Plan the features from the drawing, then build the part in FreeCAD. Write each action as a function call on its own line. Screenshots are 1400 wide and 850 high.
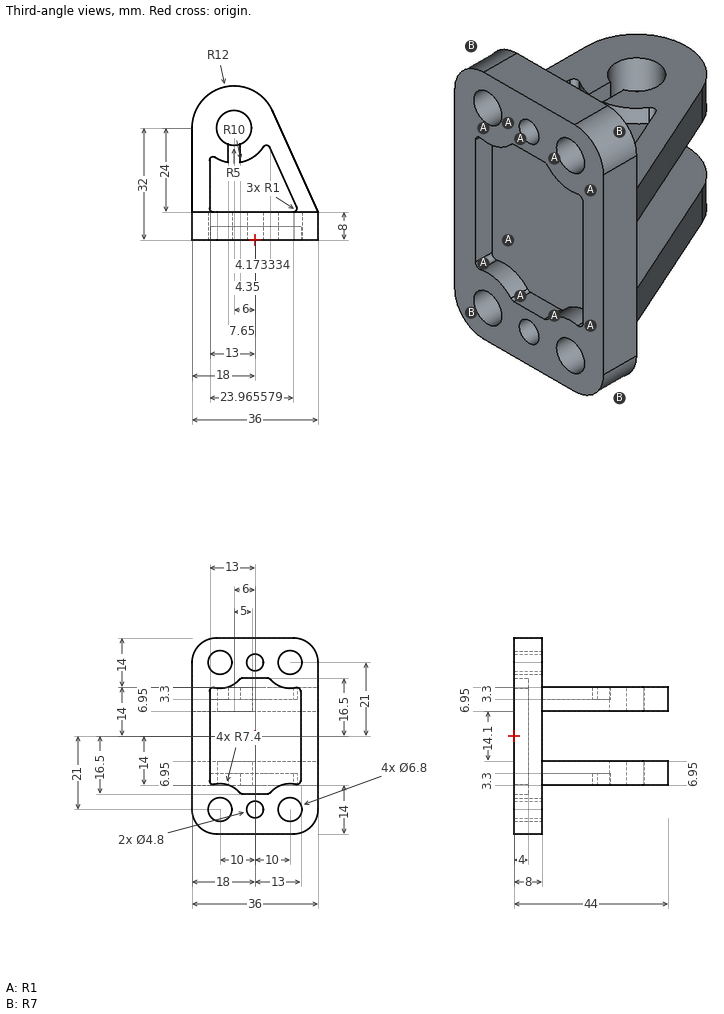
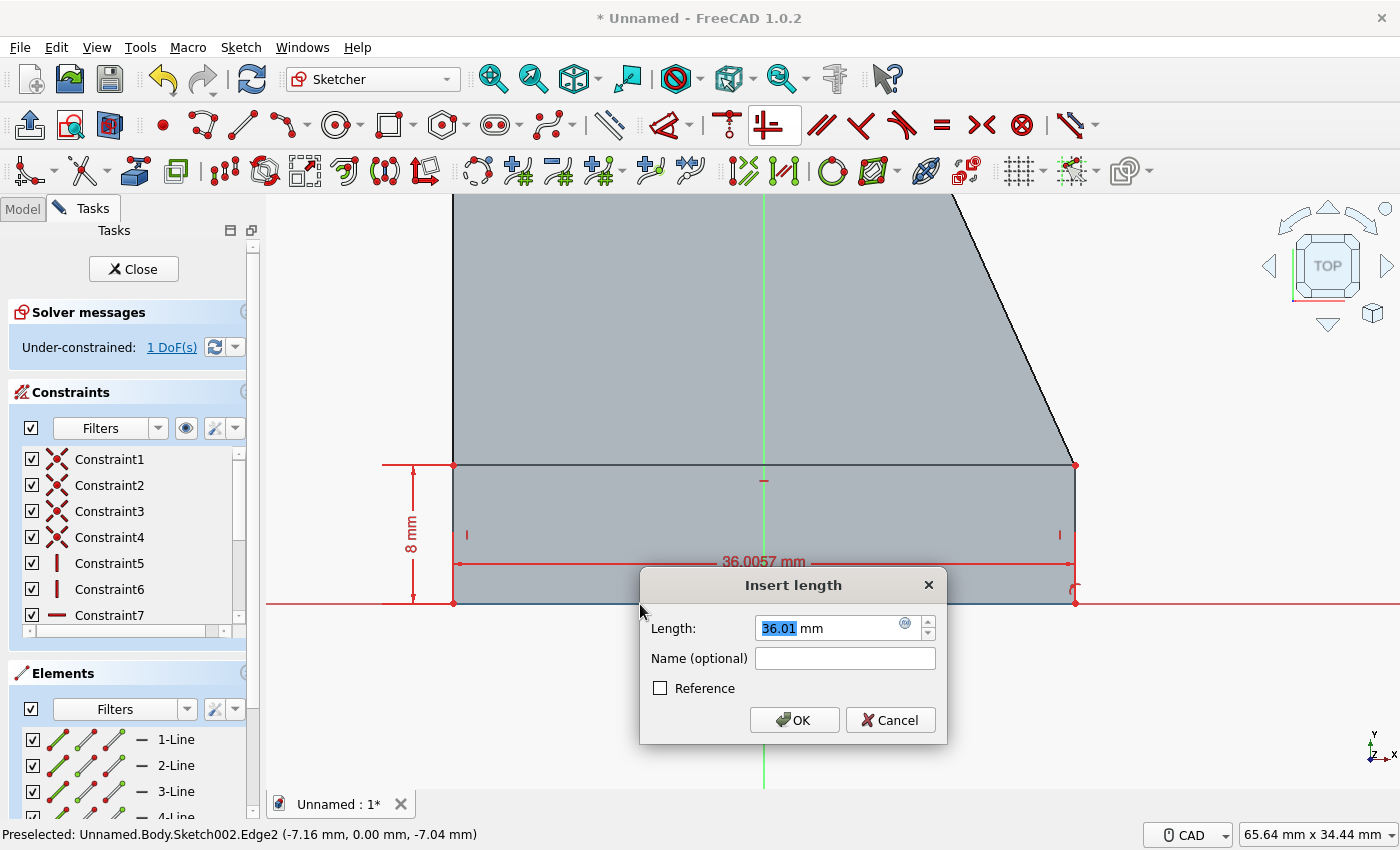
text(36)
key(Return)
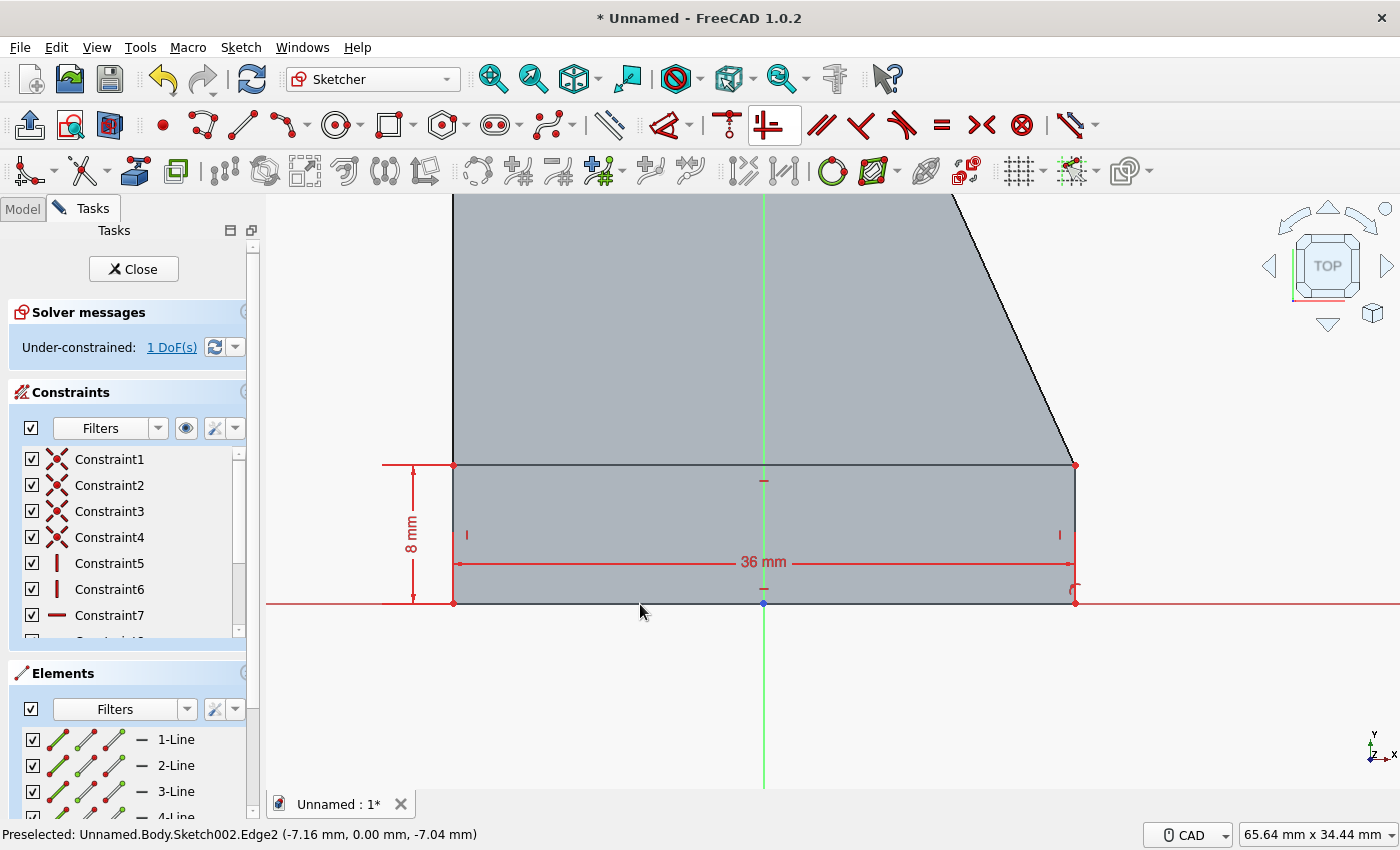
click(453, 465)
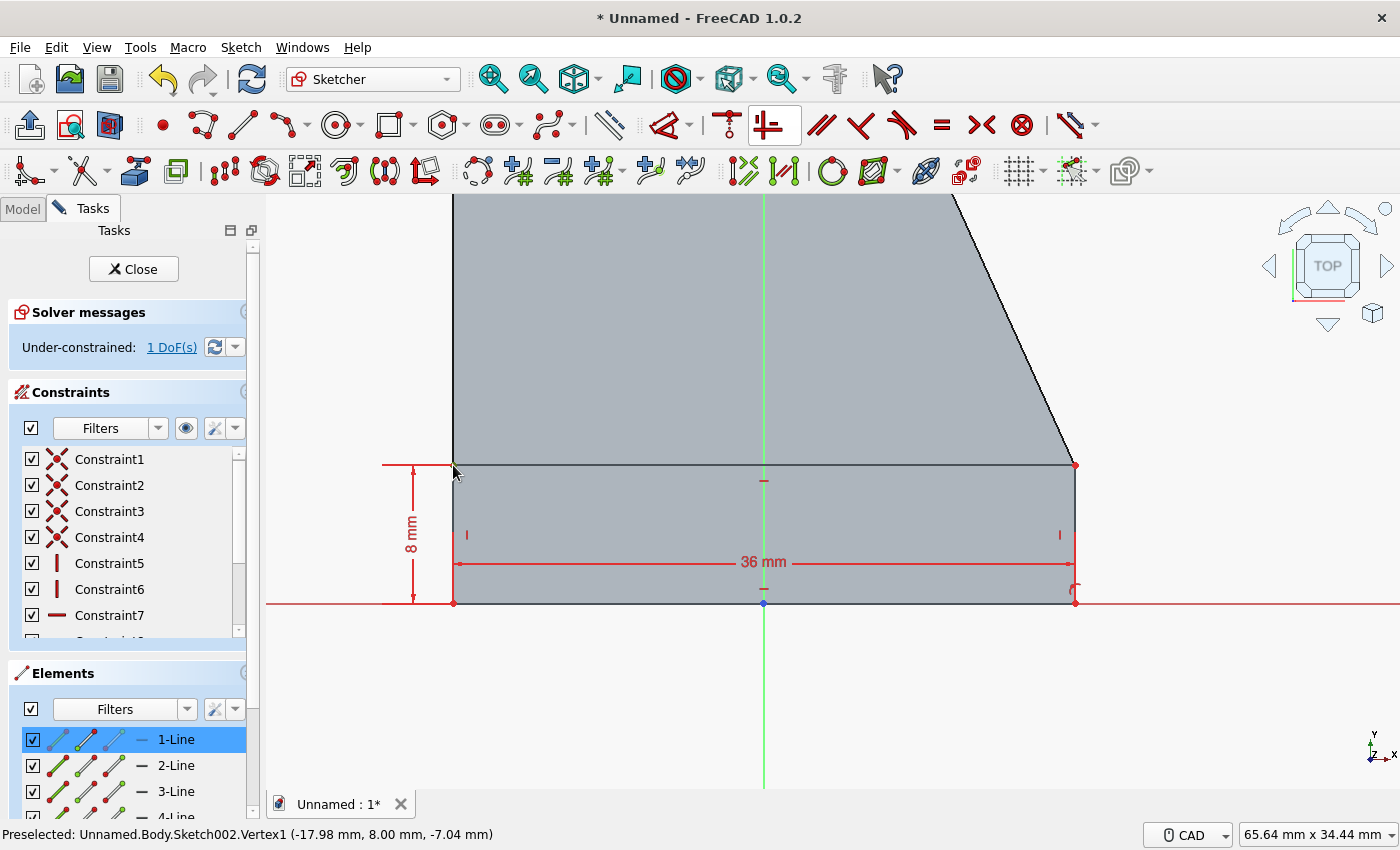
key(l)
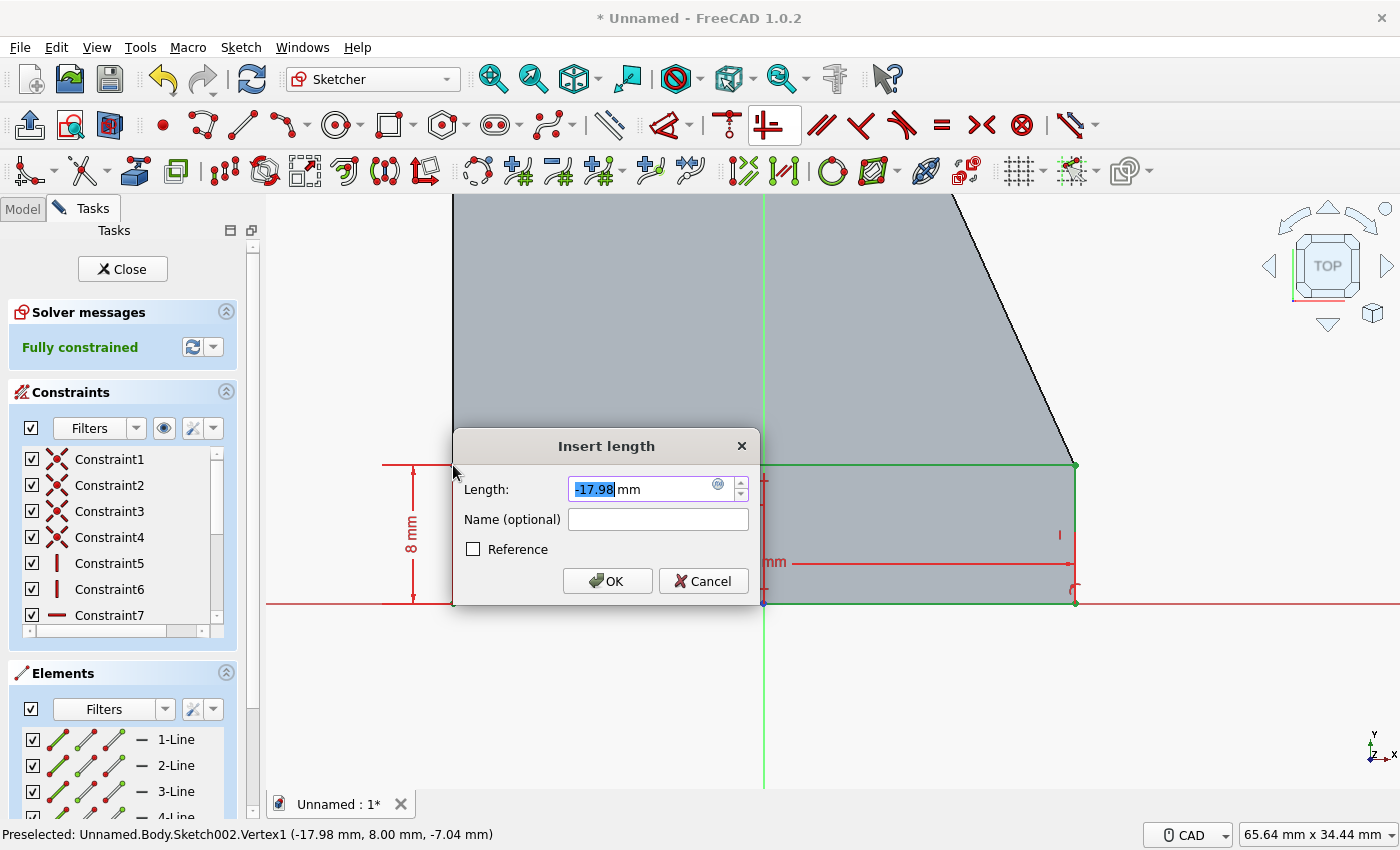
text(-18)
key(Return)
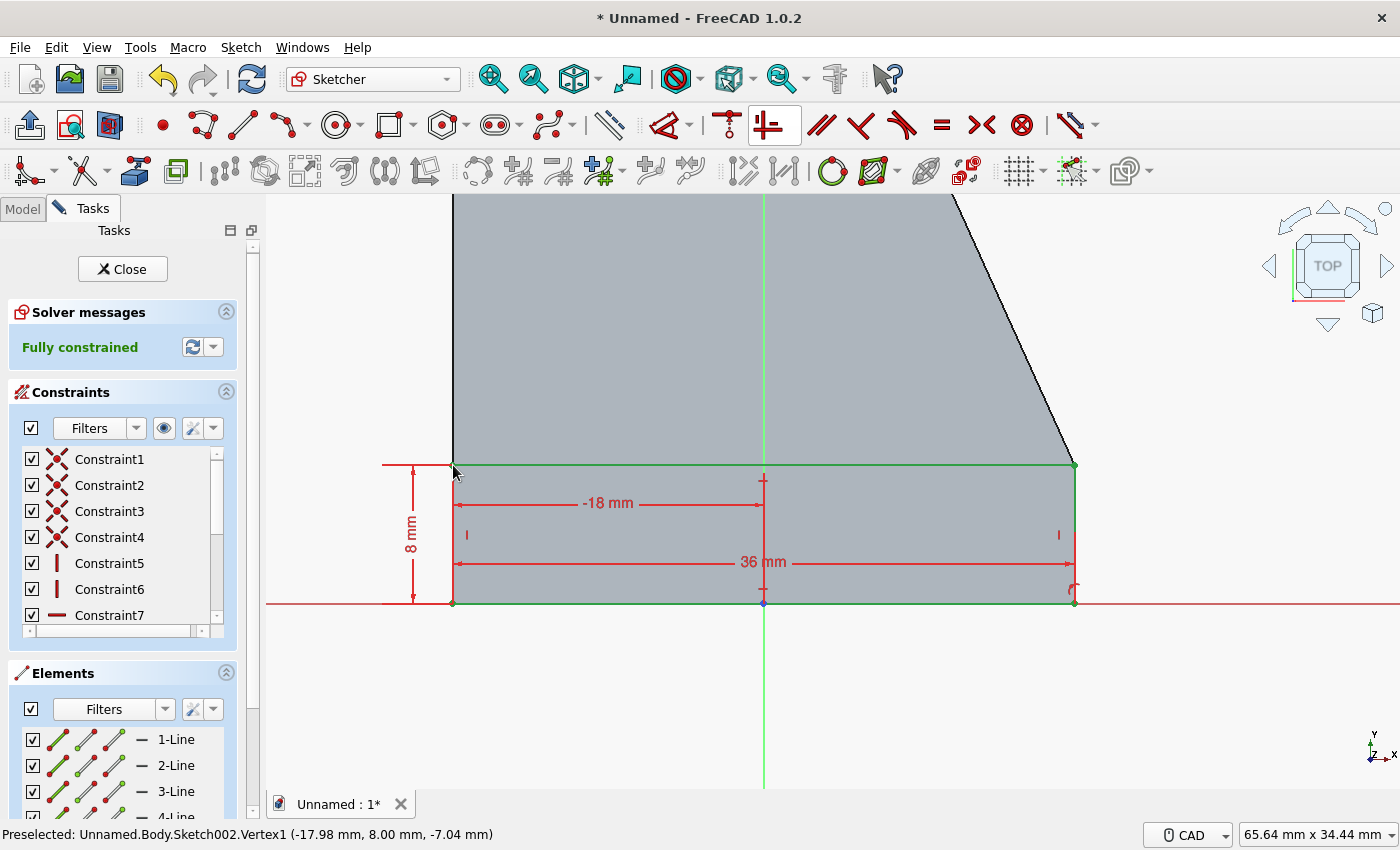
click(123, 269)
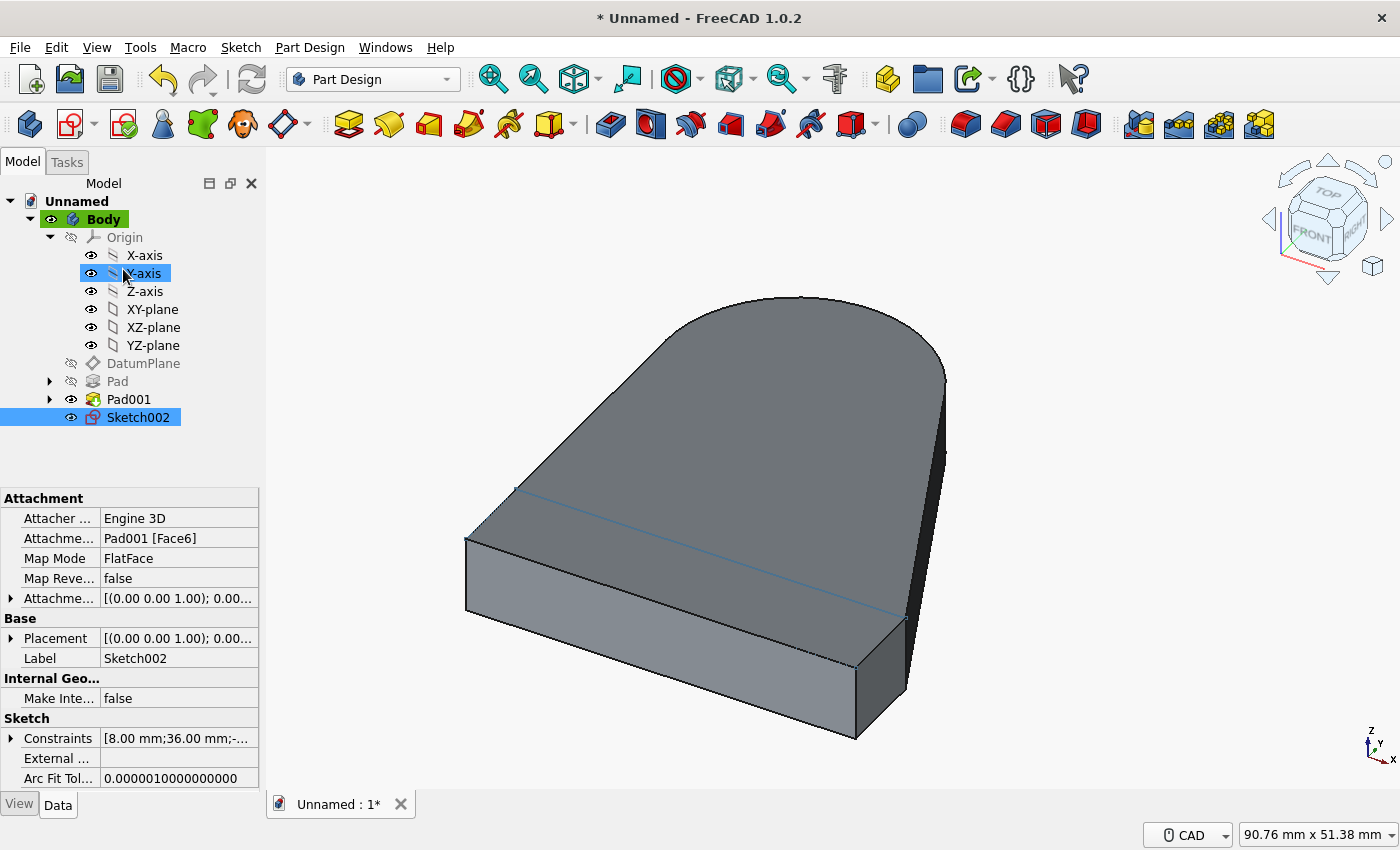
click(350, 124)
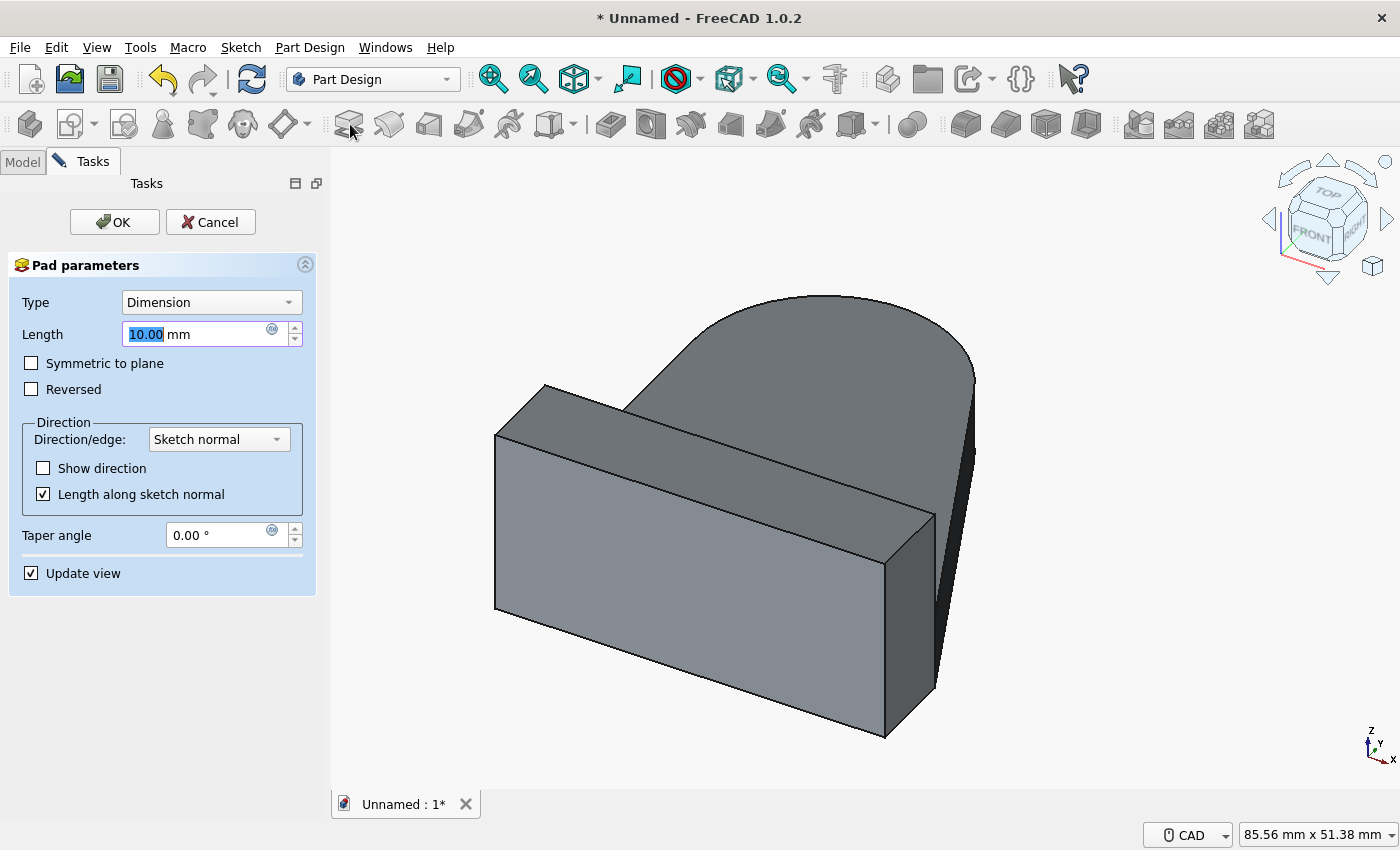
text(14.1)
key(Tab)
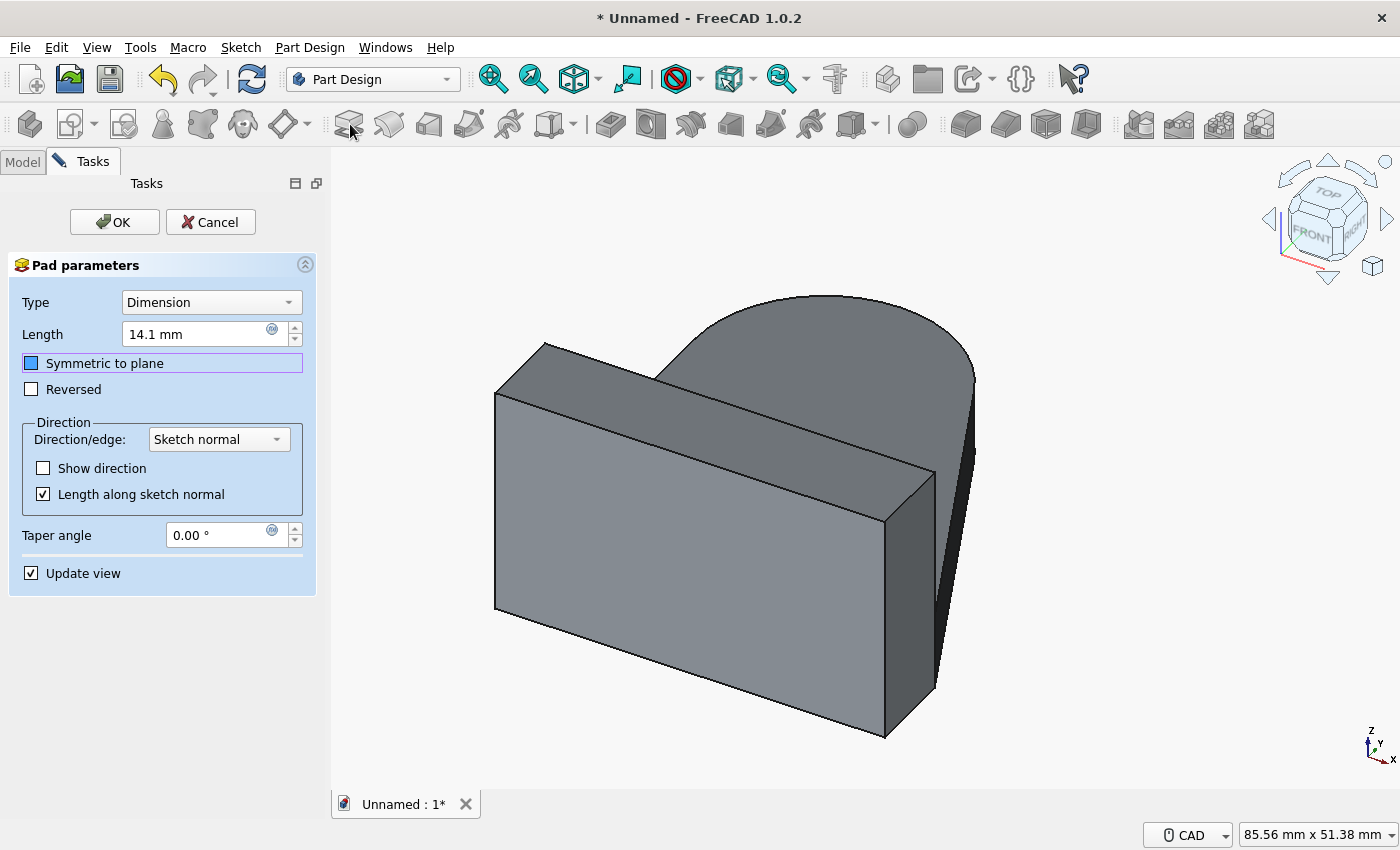
click(115, 222)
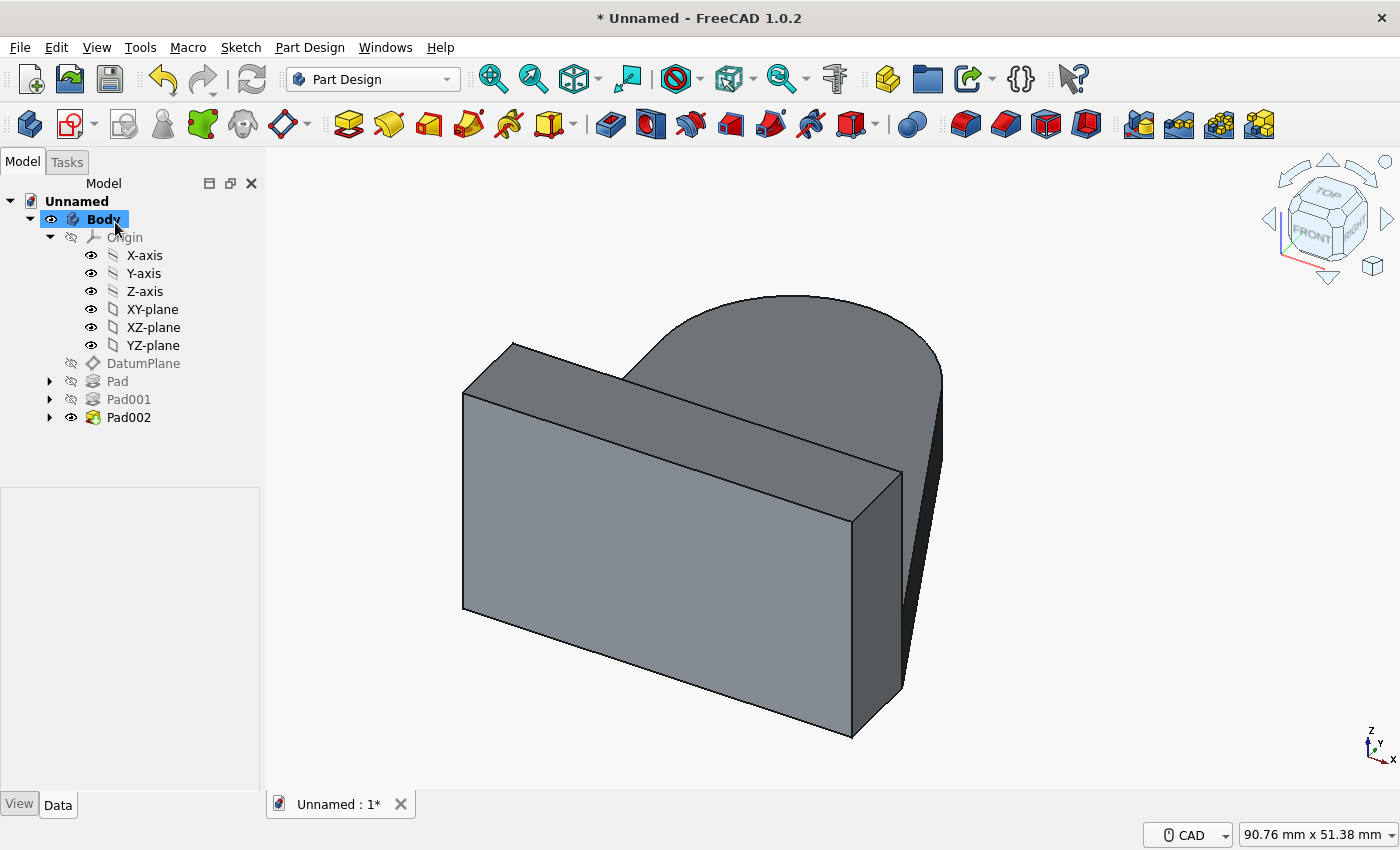
click(494, 80)